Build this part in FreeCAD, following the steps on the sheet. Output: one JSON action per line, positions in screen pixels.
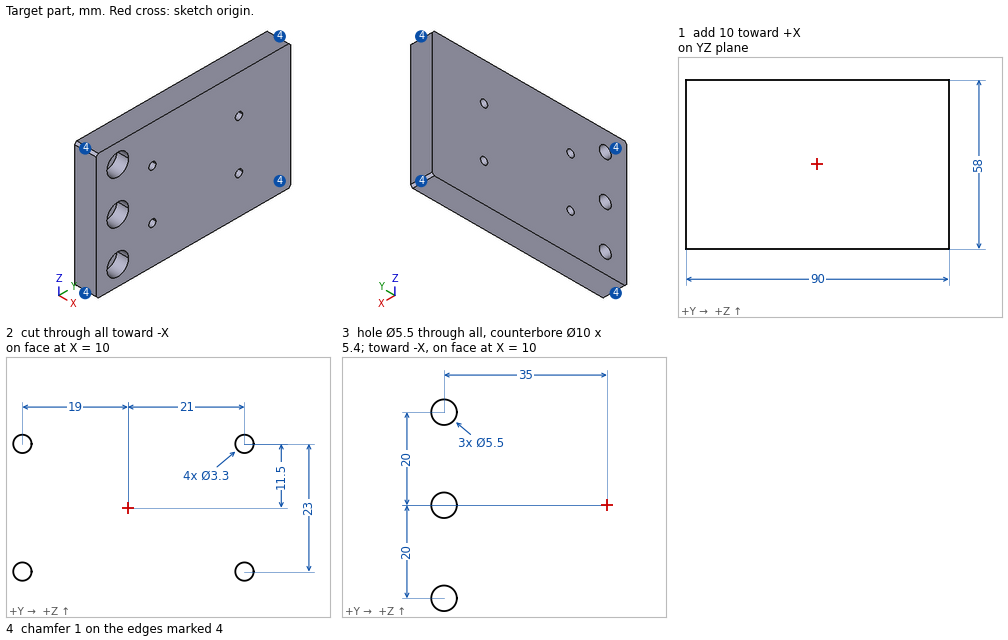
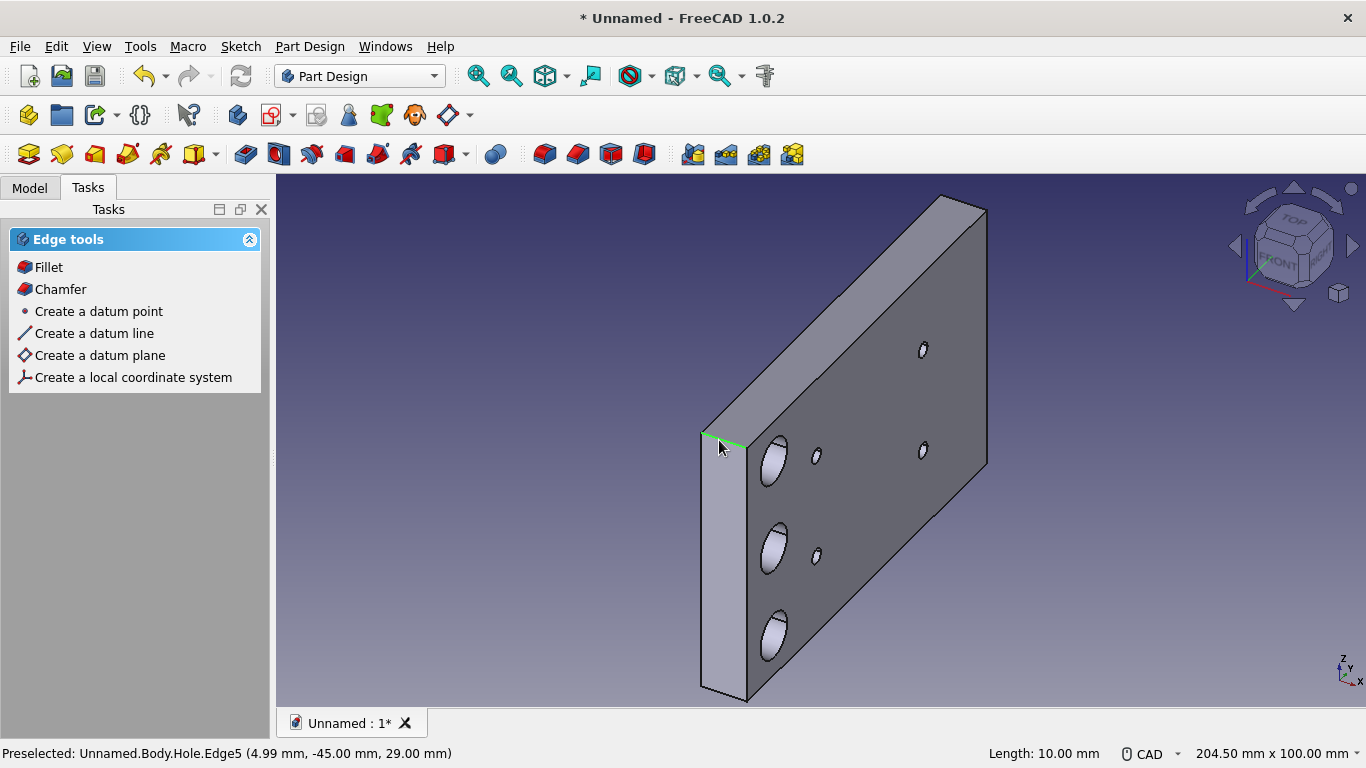
{"action": "key", "text": "0"}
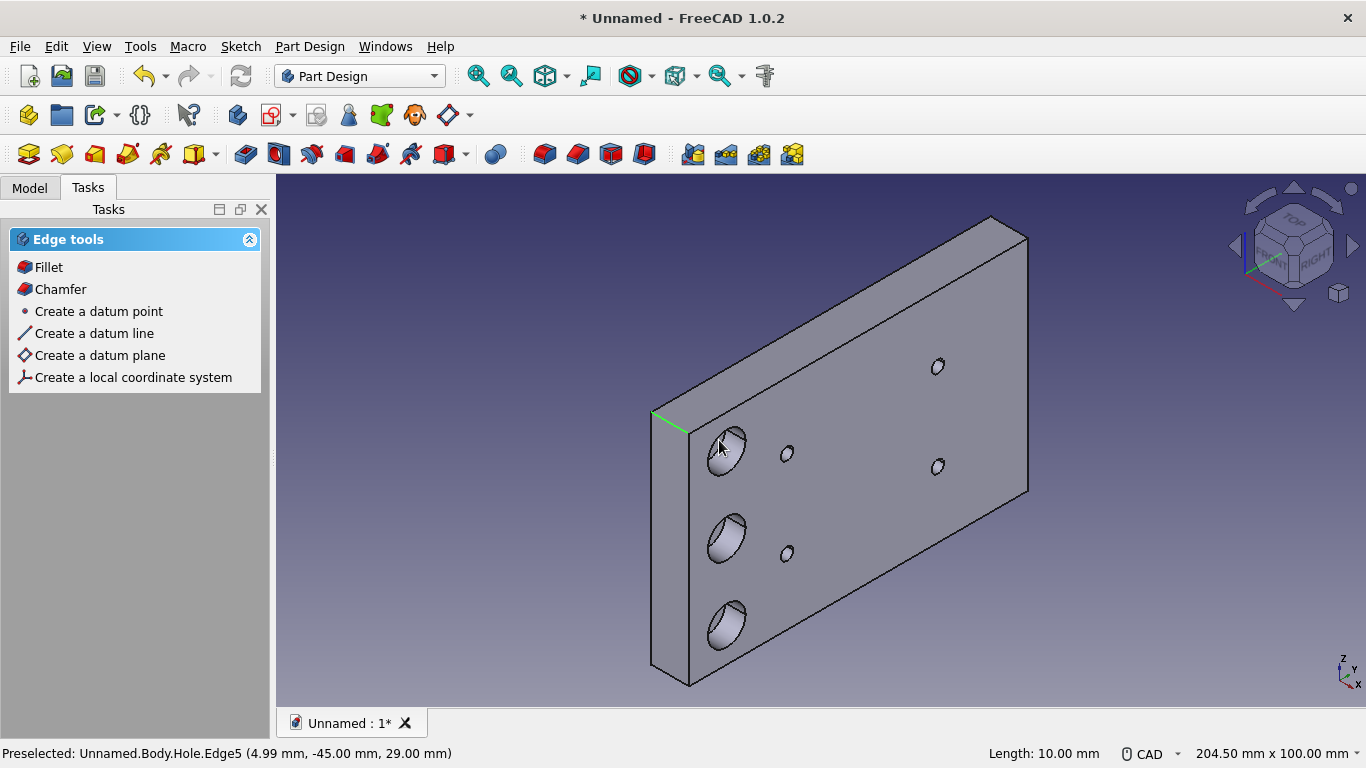
{"action": "key", "text": "2"}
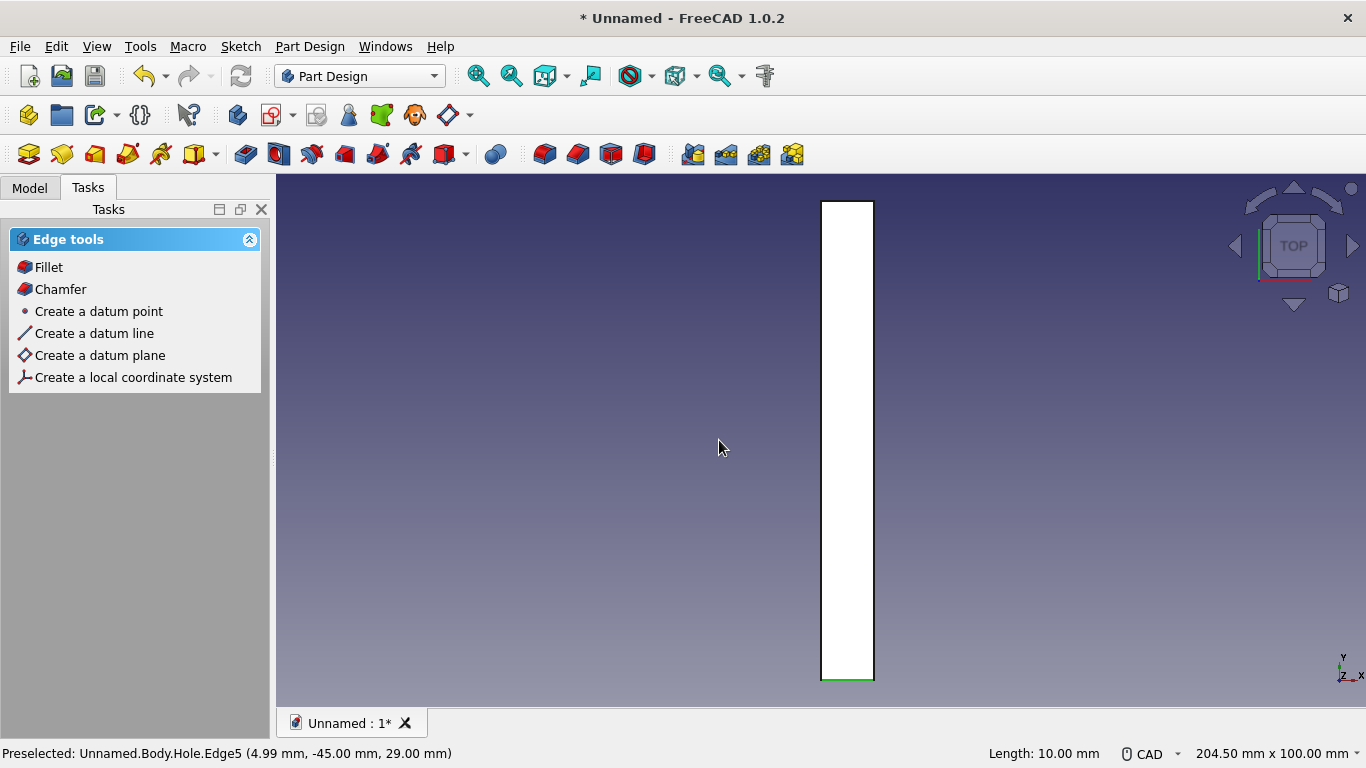
{"action": "key", "text": "1"}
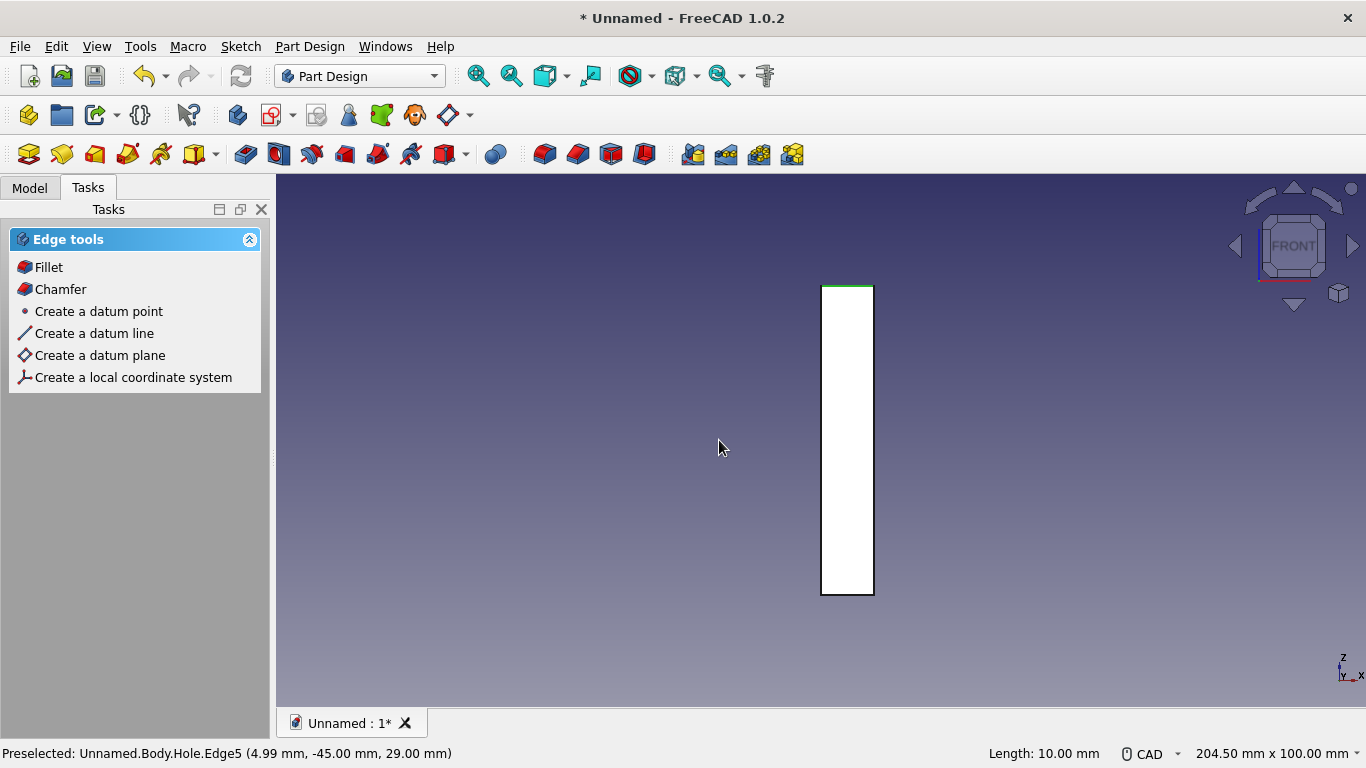
{"action": "left_click", "coordinate": [848, 594], "text": "ctrl"}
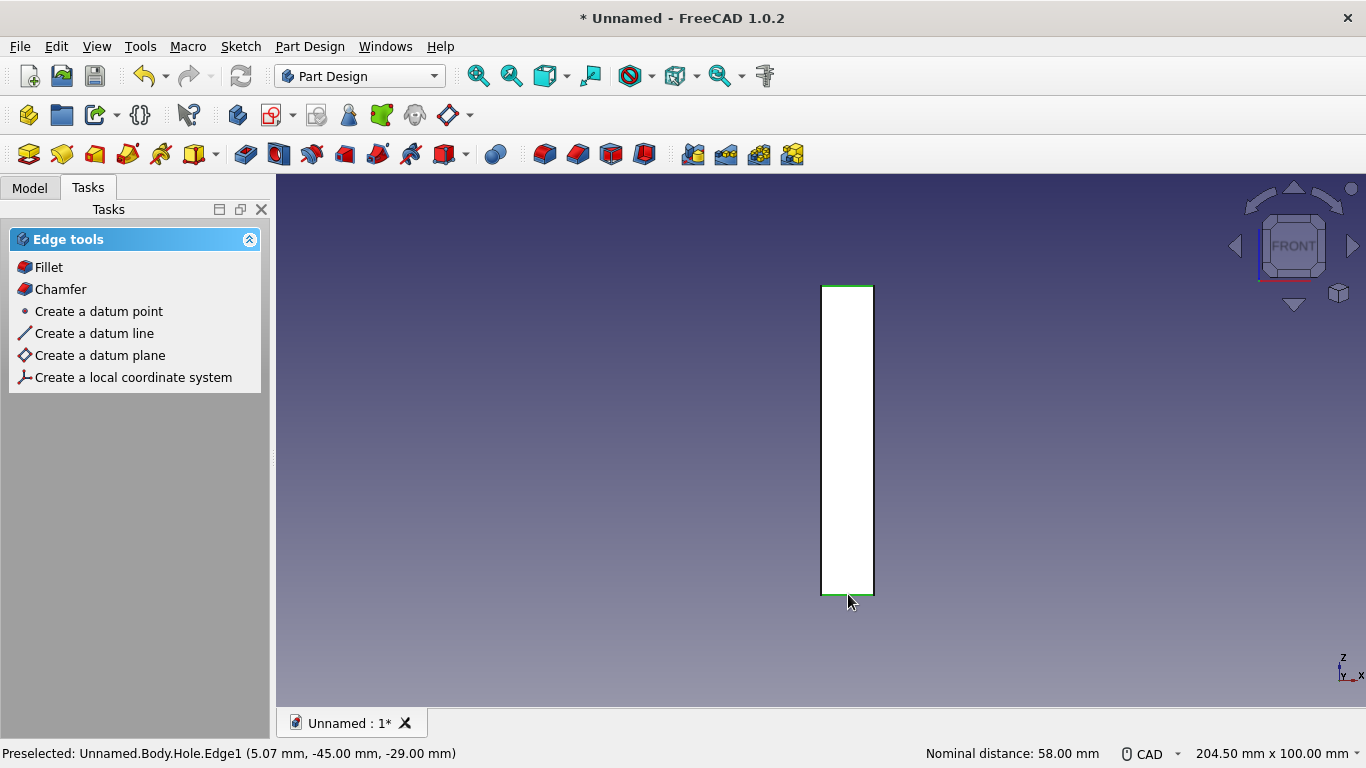
{"action": "key", "text": "3"}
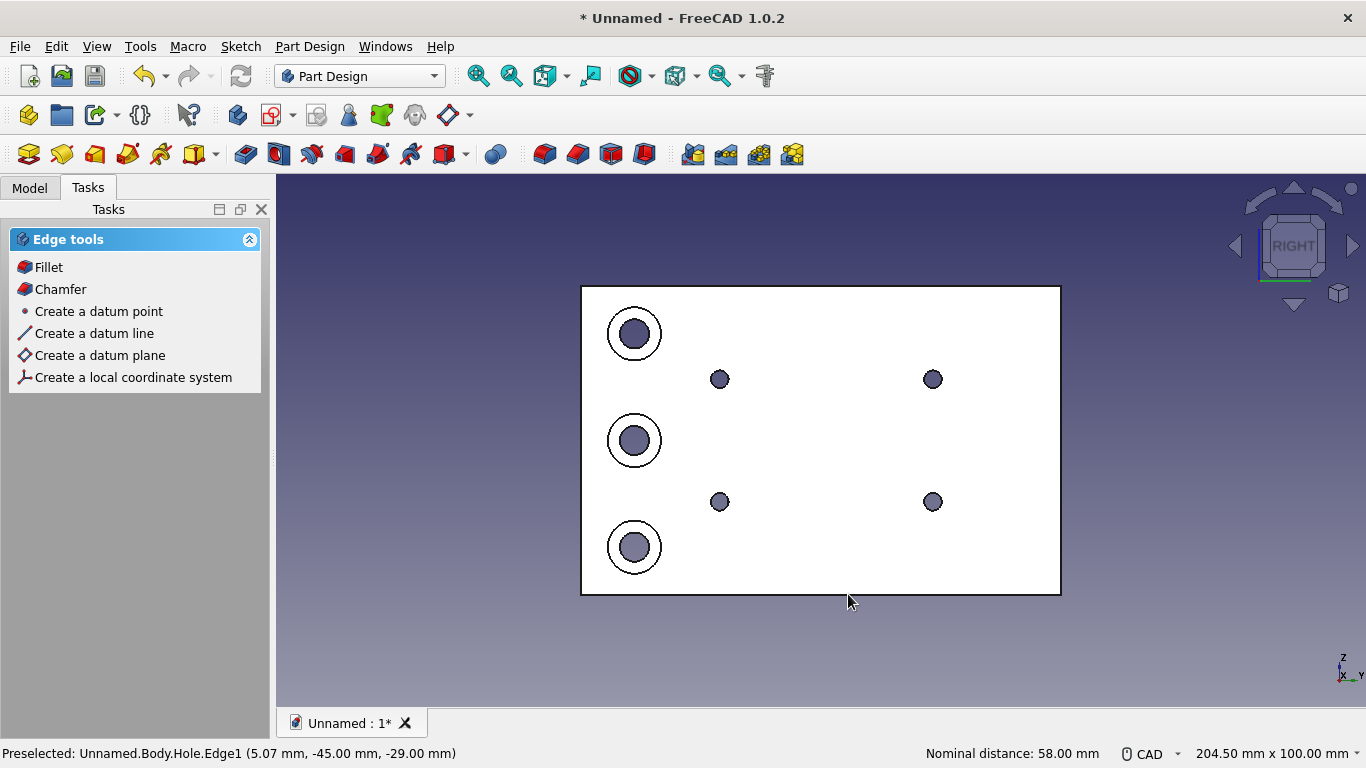
{"action": "key", "text": "5"}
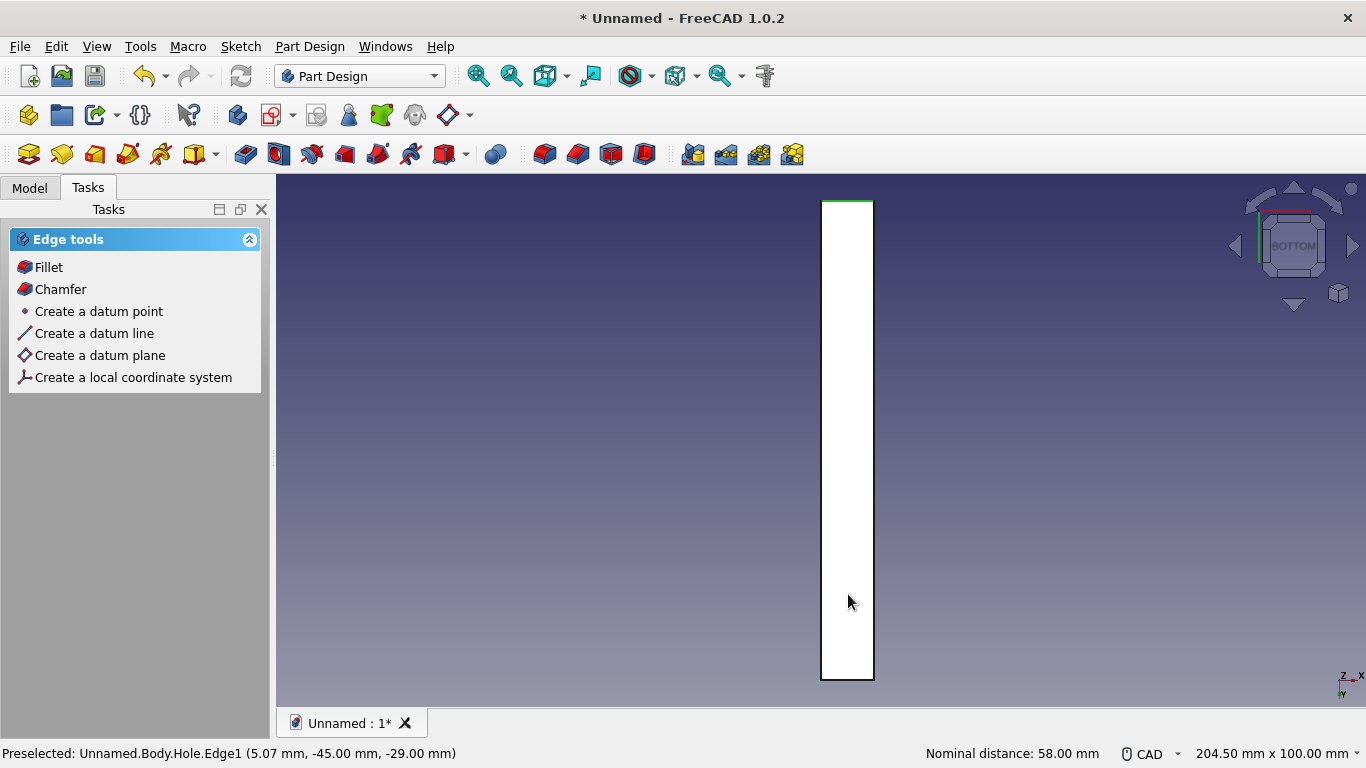
{"action": "key", "text": "4"}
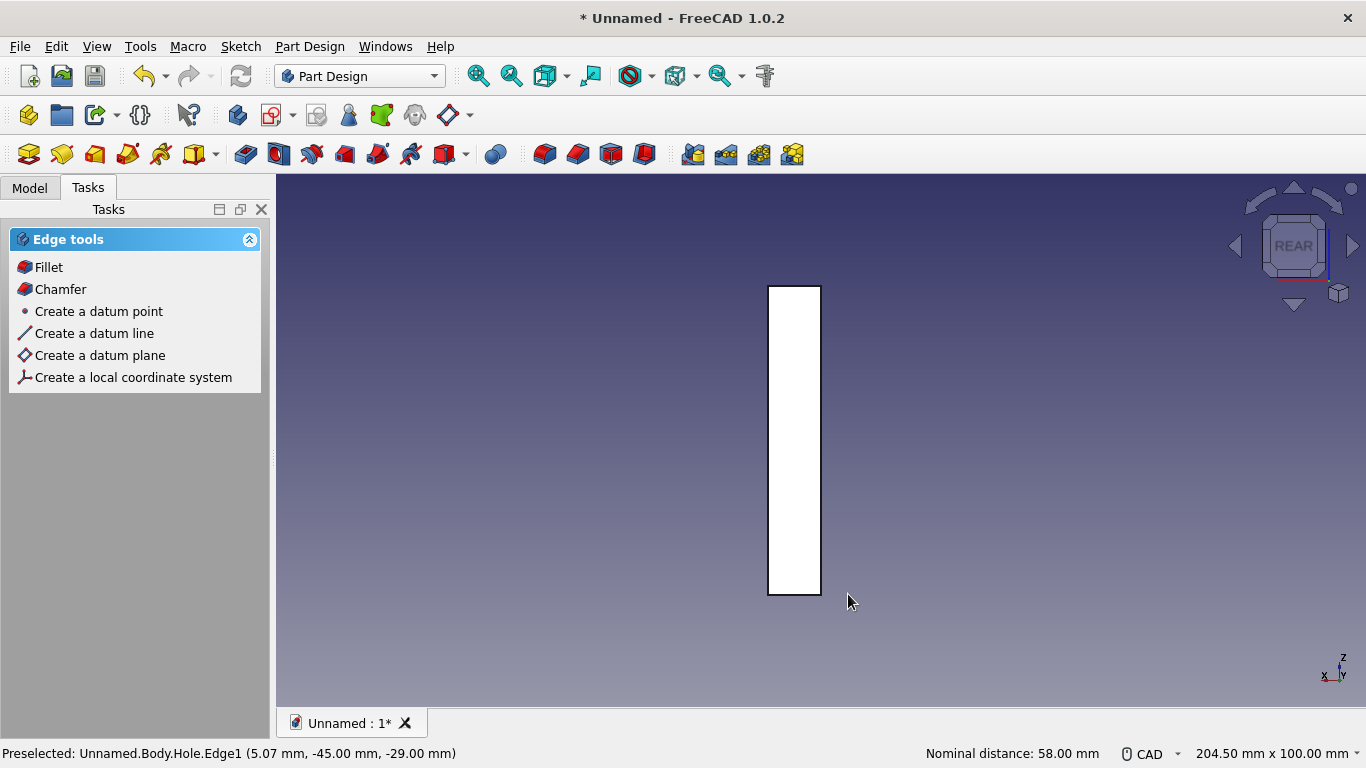
{"action": "left_click", "coordinate": [794, 285], "text": "ctrl"}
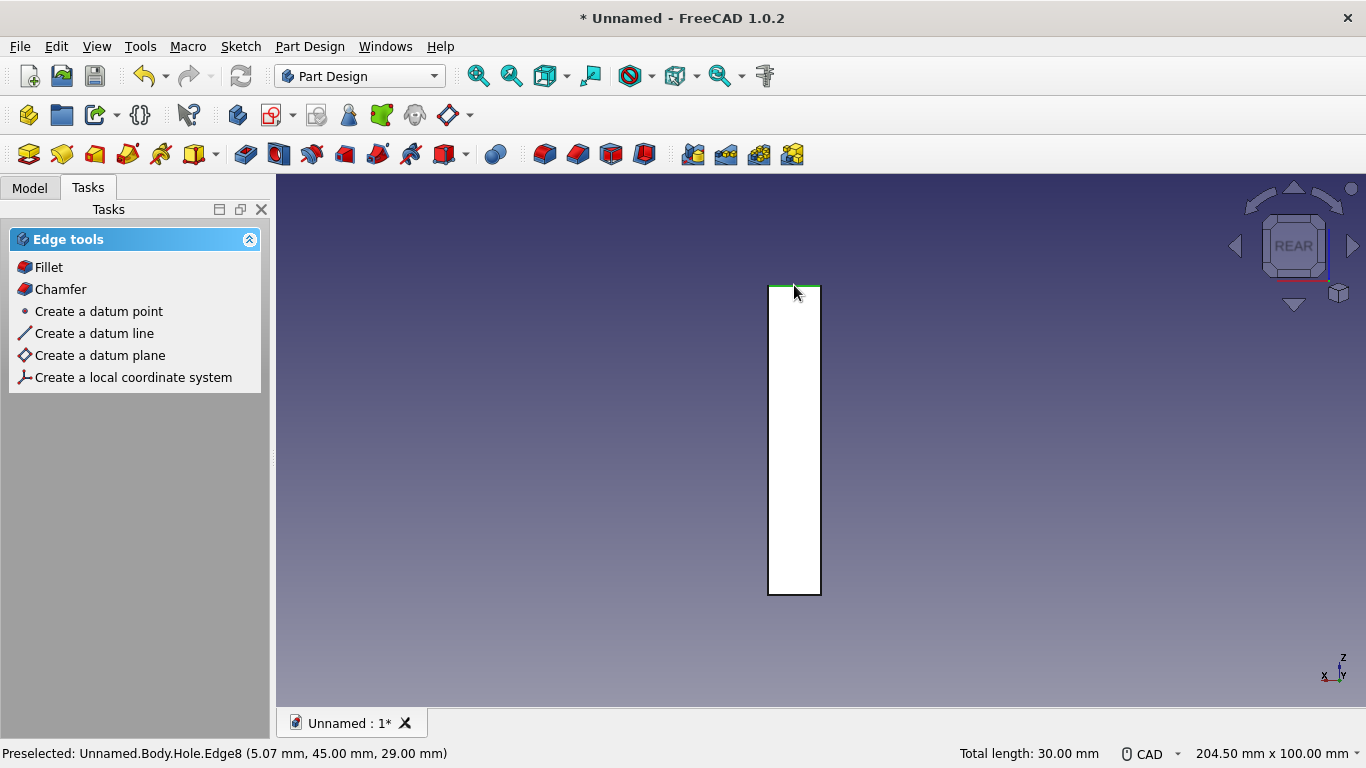
{"action": "left_click", "coordinate": [794, 594], "text": "ctrl"}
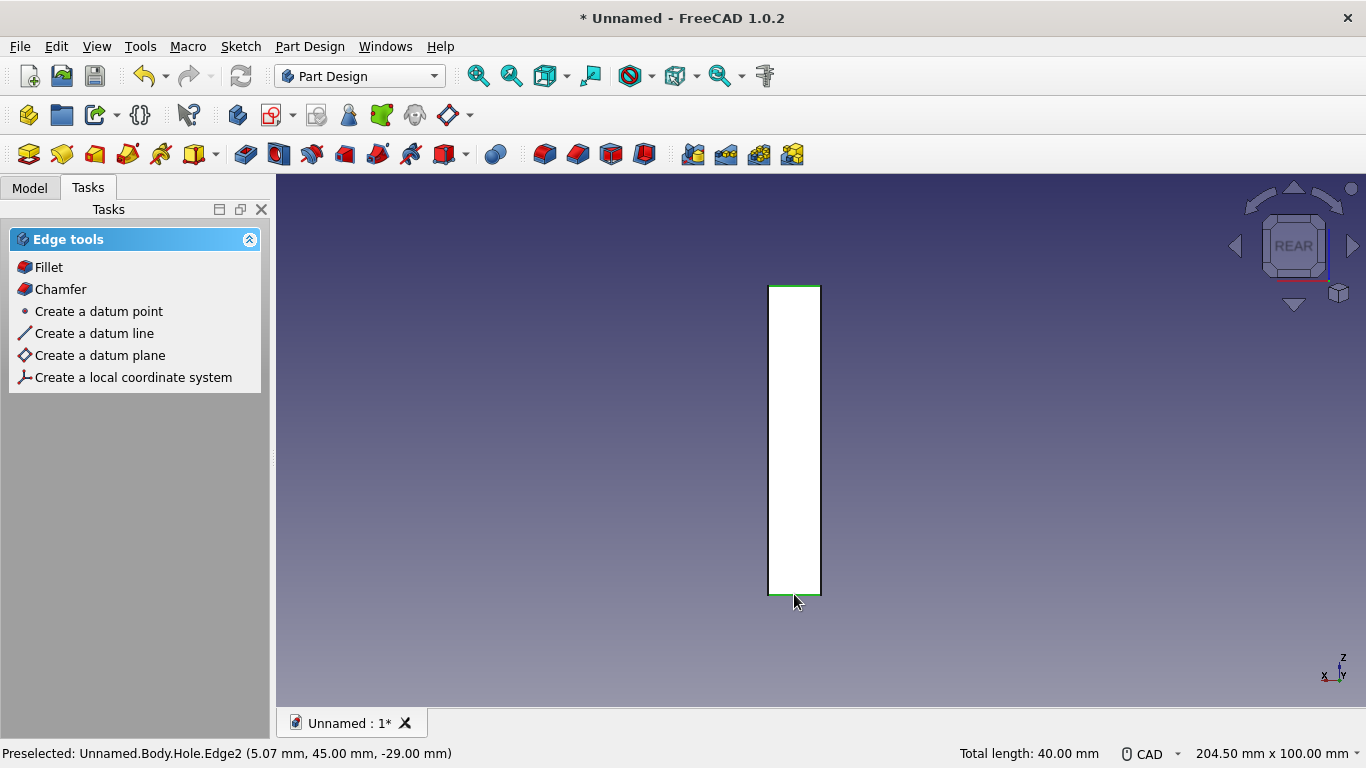
{"action": "left_click", "coordinate": [578, 154]}